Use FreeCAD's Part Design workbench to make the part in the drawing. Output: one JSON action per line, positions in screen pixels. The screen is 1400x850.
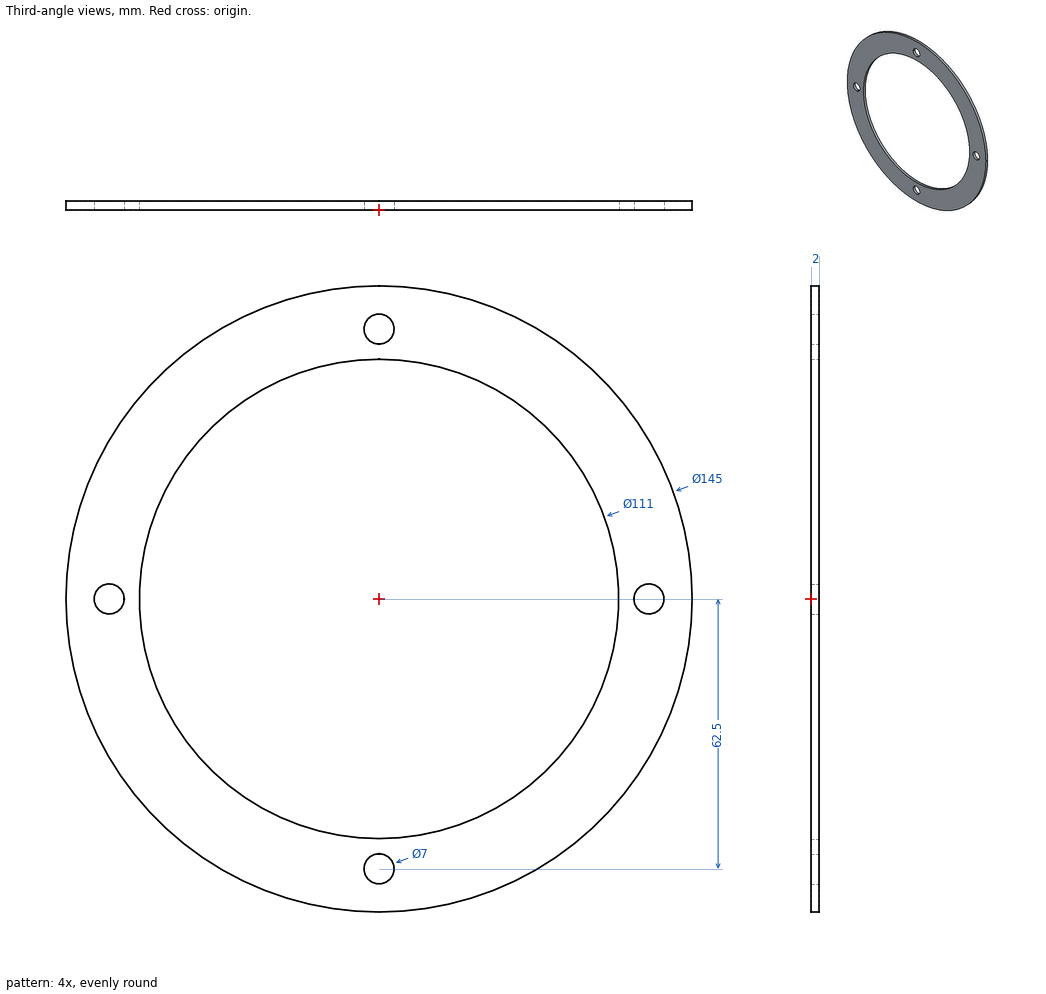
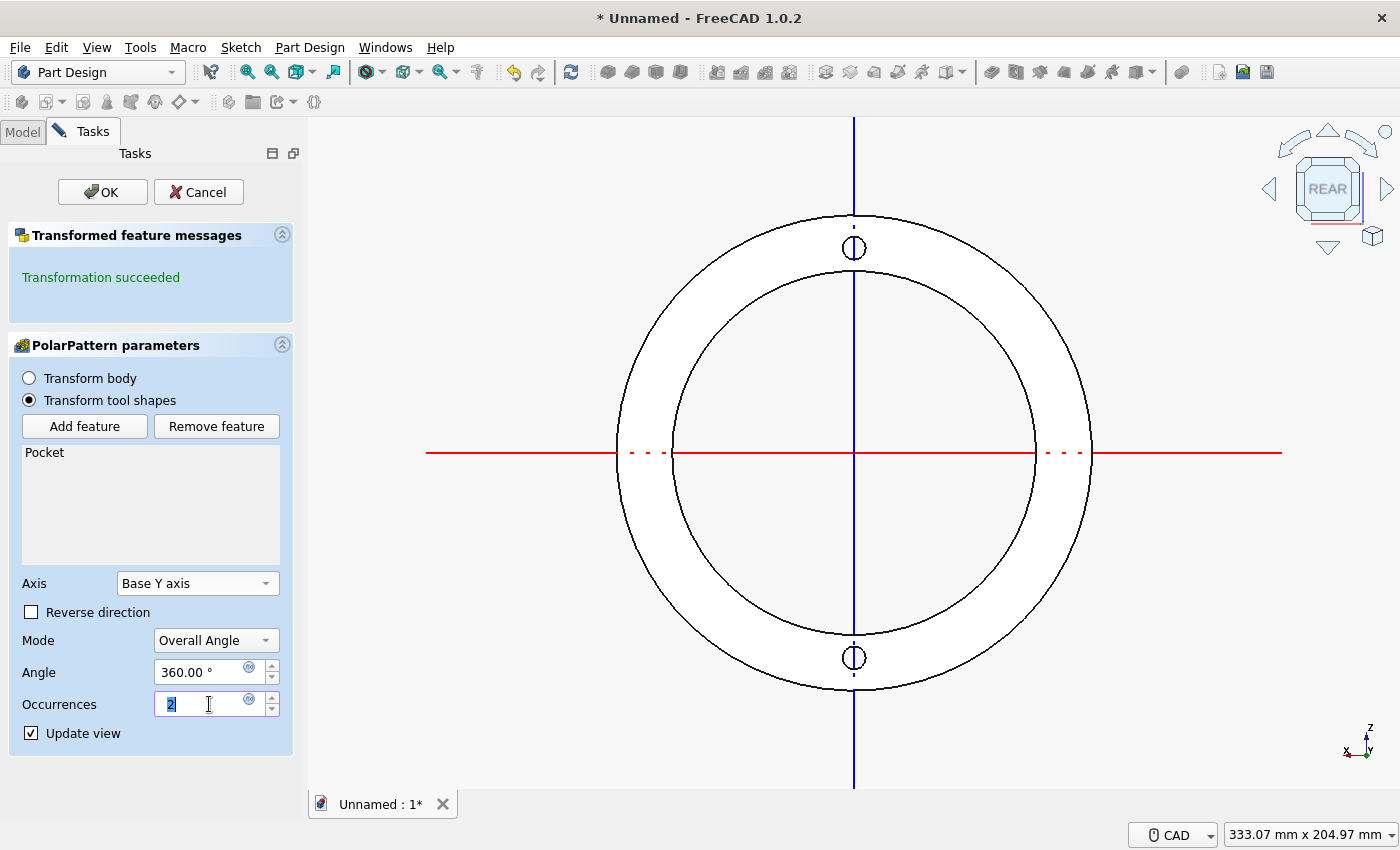
{"action": "type", "text": "4"}
{"action": "key", "text": "Tab"}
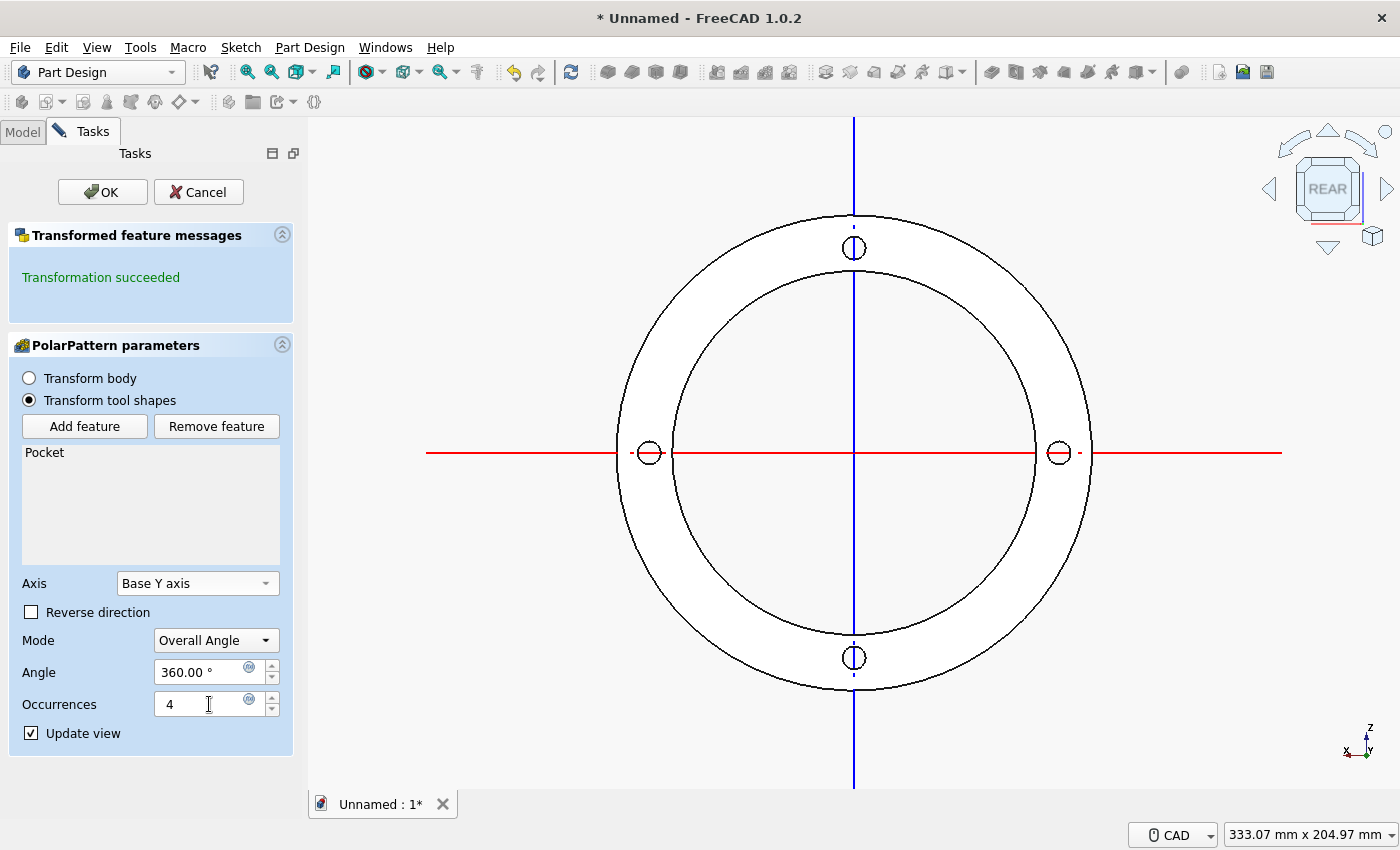
{"action": "left_click", "coordinate": [103, 192]}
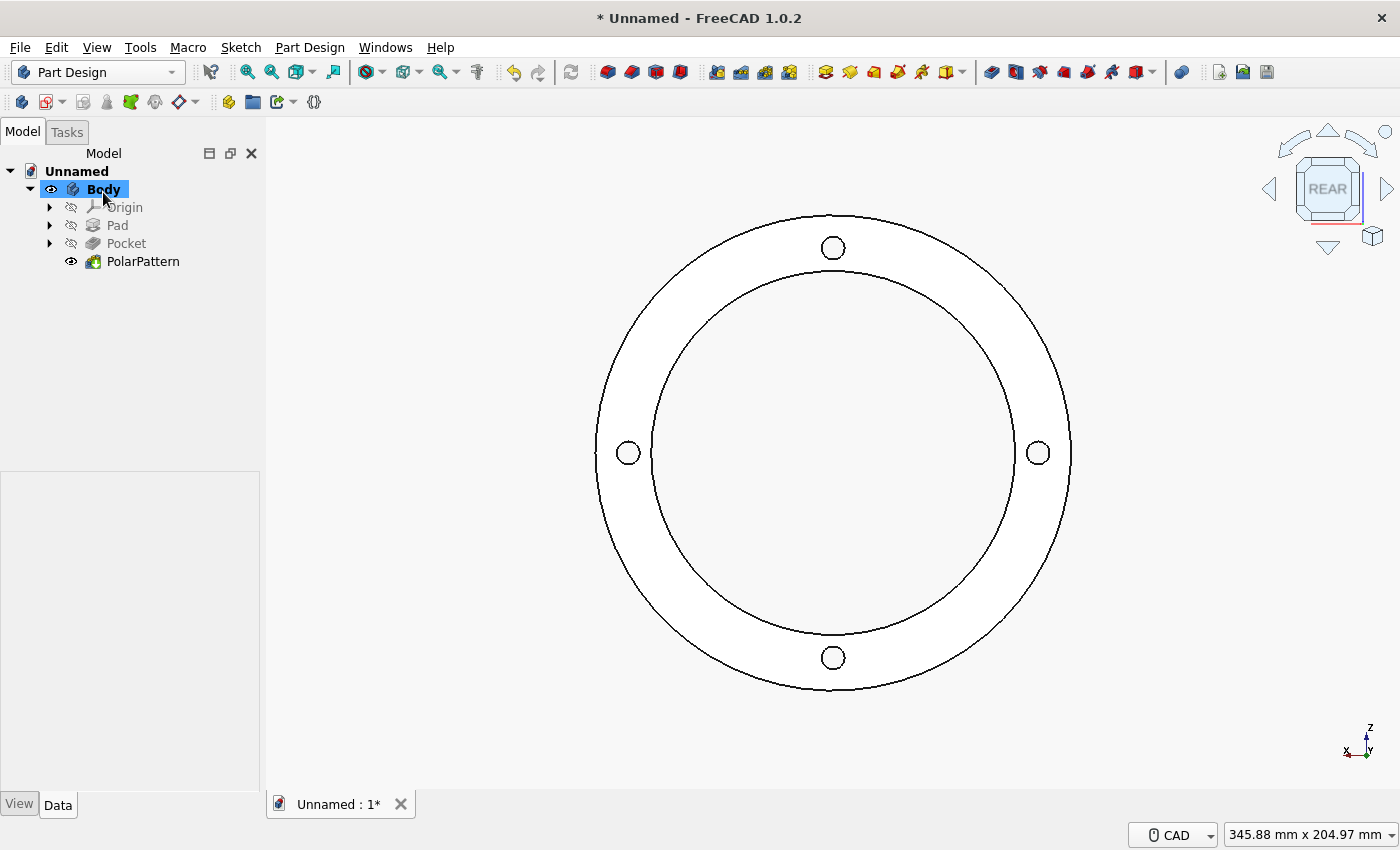
{"action": "key", "text": "0"}